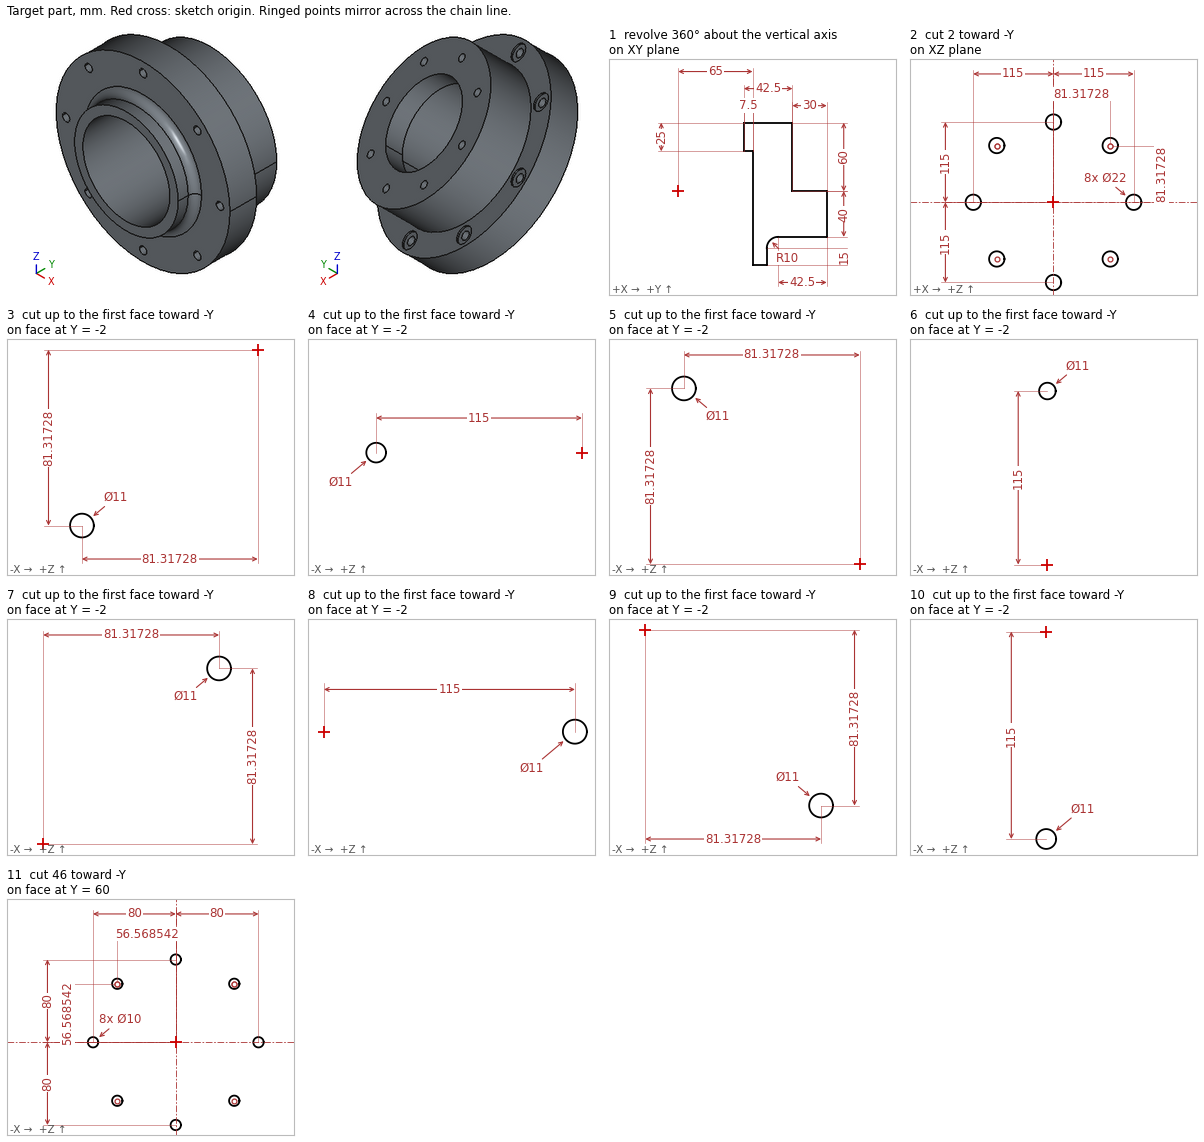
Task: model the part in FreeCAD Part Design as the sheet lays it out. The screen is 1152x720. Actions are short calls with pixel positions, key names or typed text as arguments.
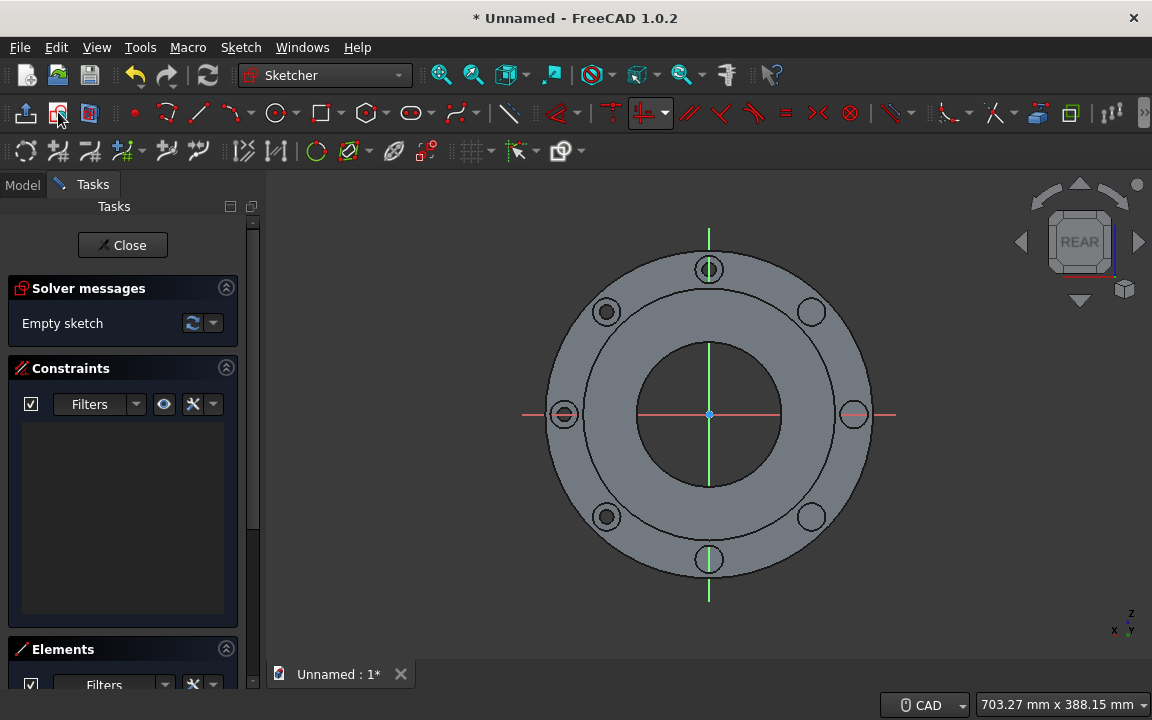
click(90, 114)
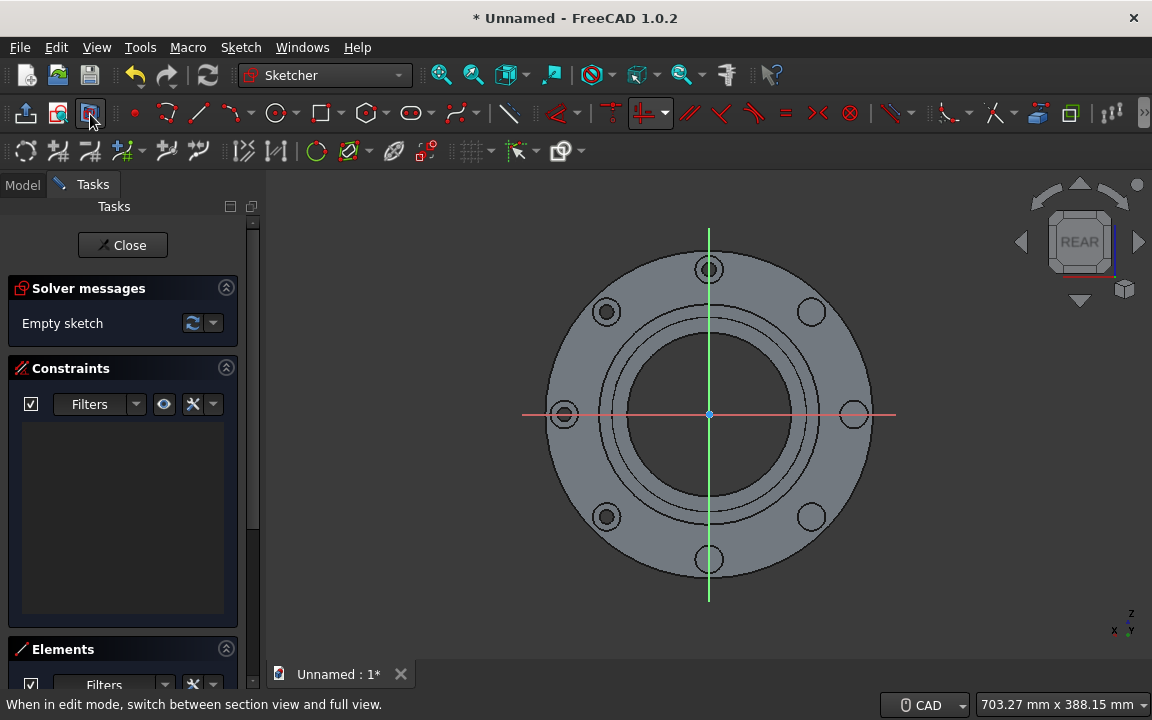
scroll(821, 307, up, 15)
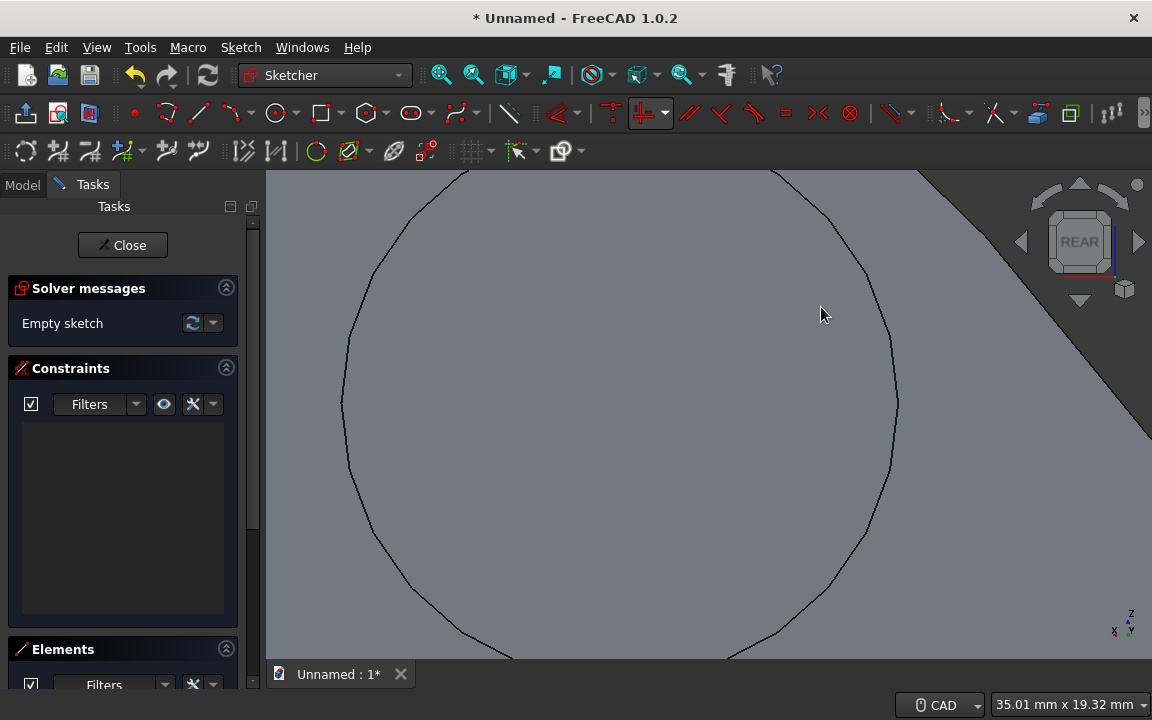
key(g)
key(c)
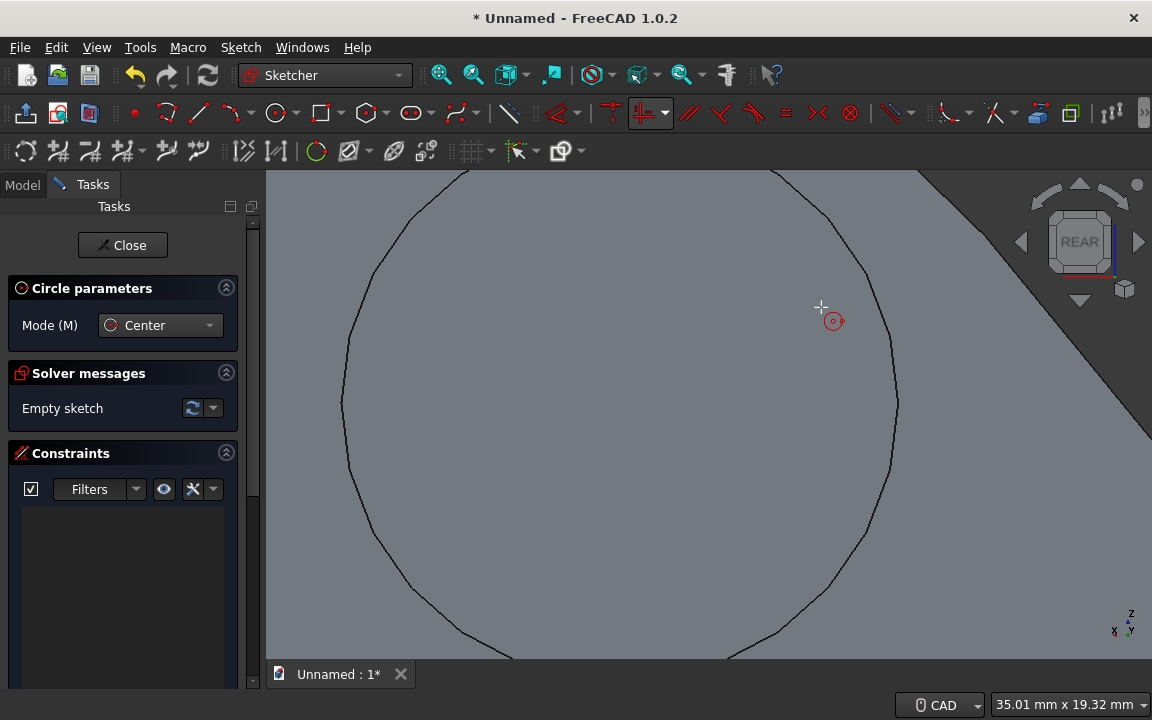
click(620, 403)
move(718, 305)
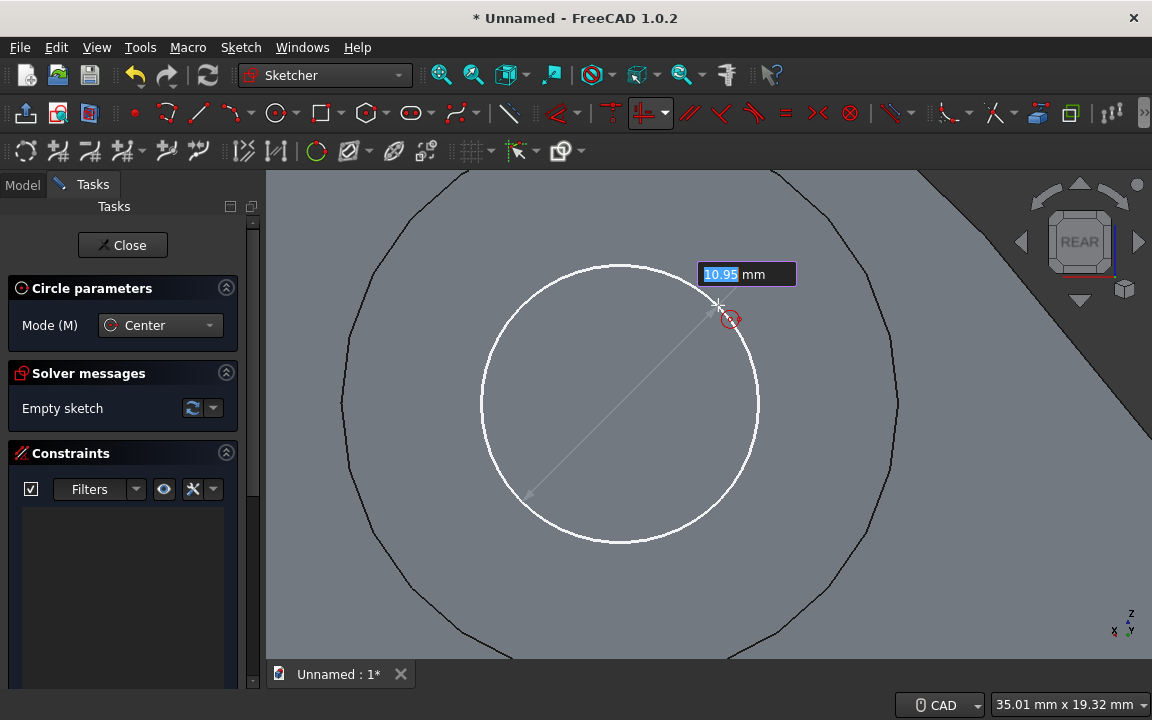
text(11)
key(Return)
key(Escape)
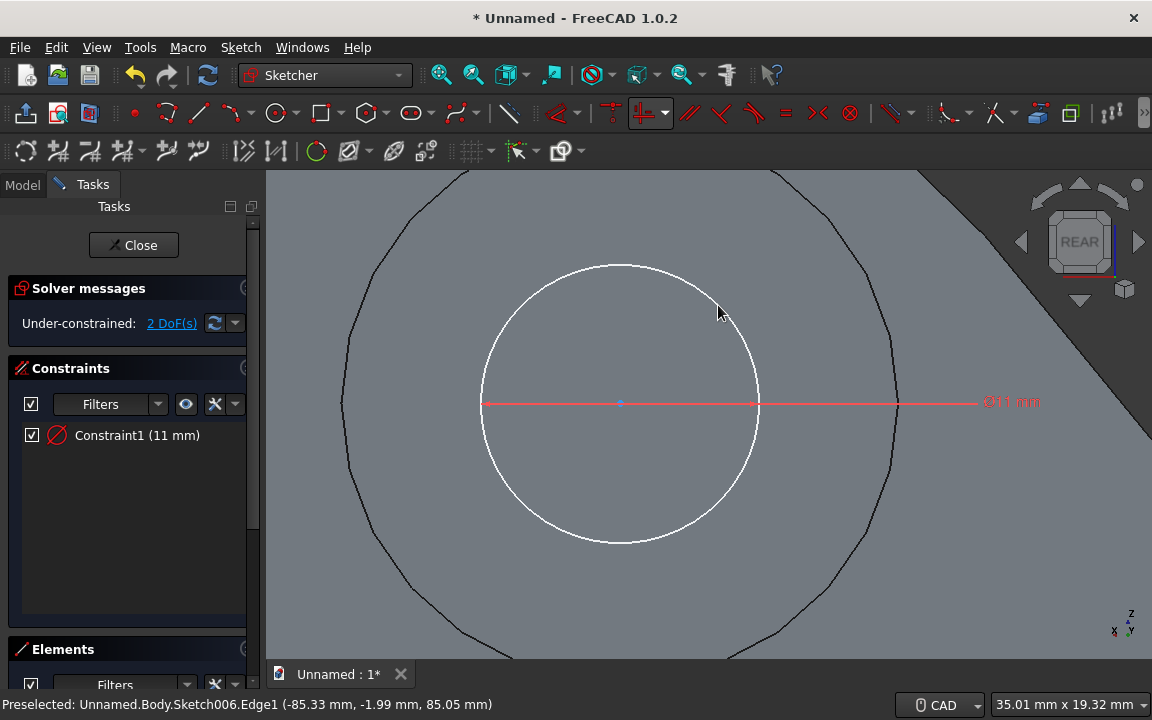
click(556, 114)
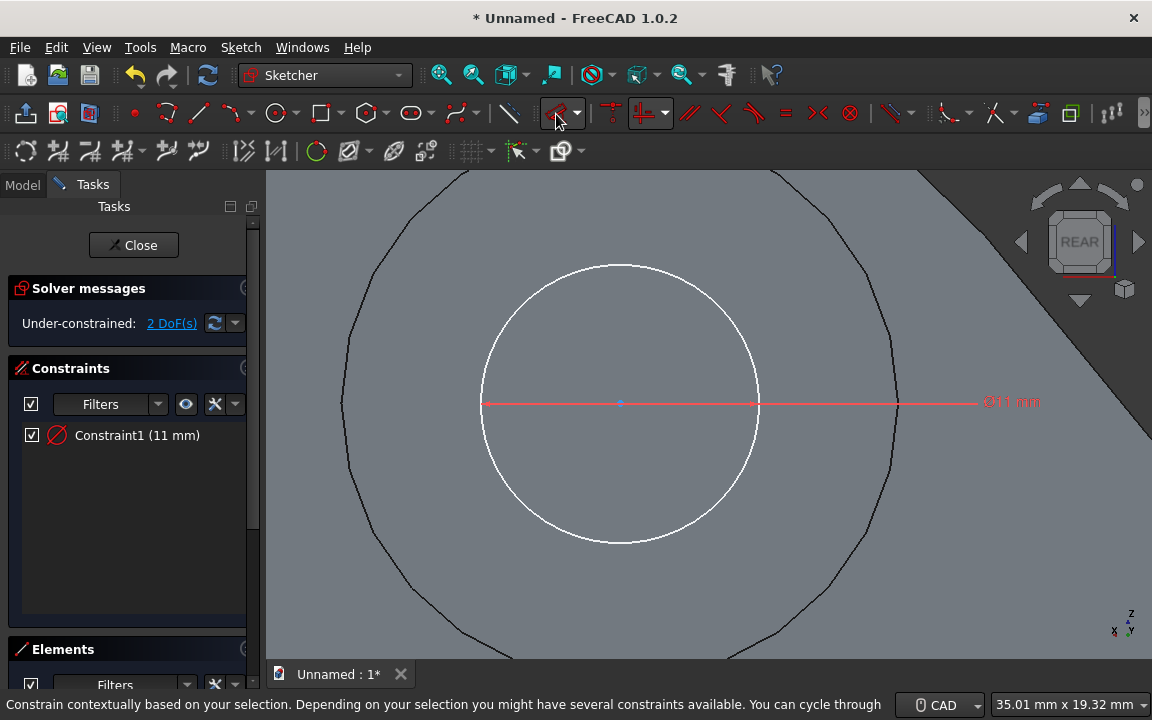
click(620, 404)
click(457, 370)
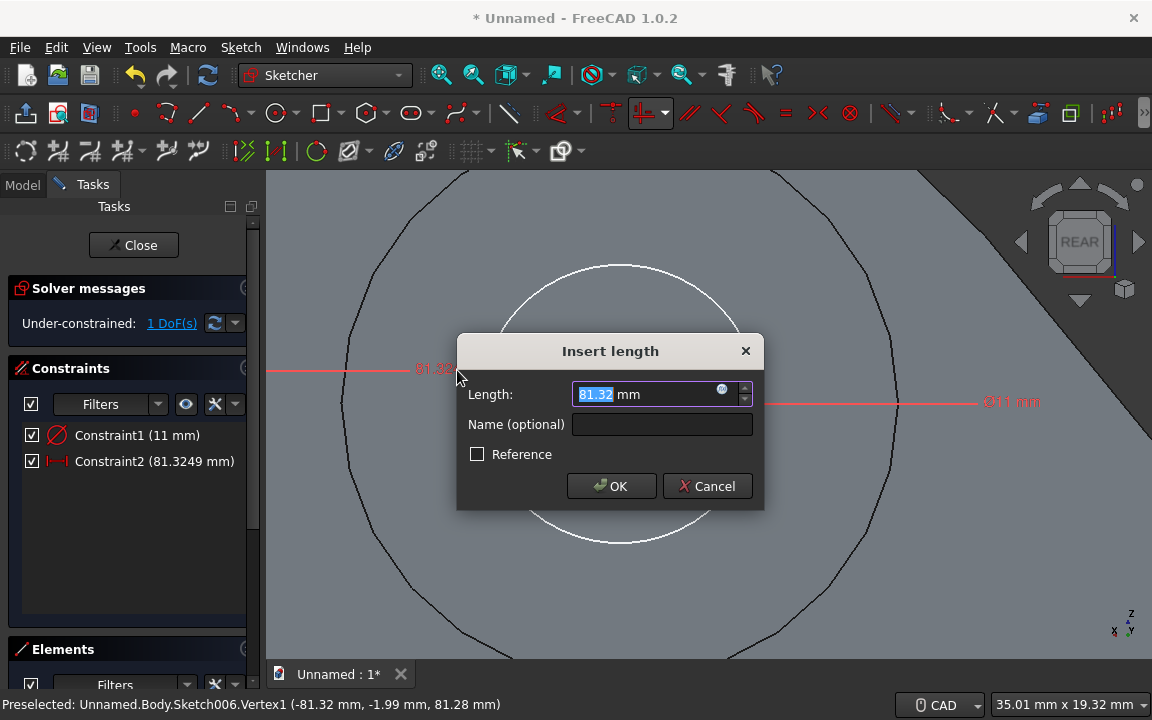
text(81.31728)
key(Return)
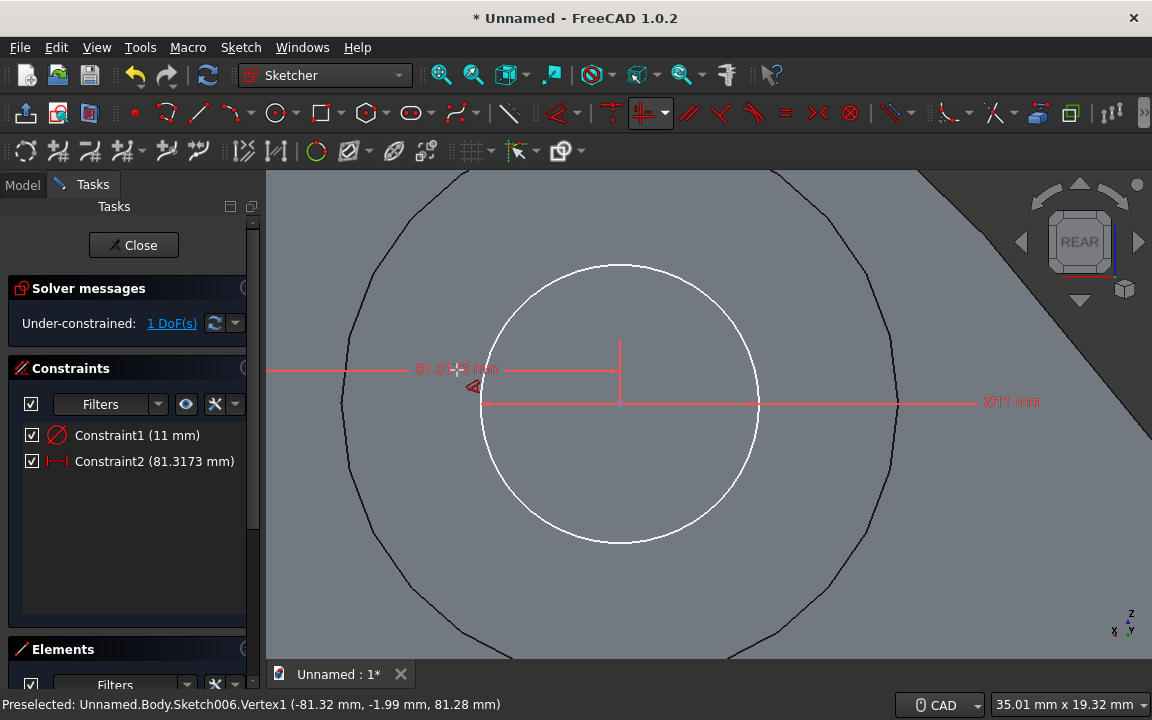
click(620, 404)
click(654, 518)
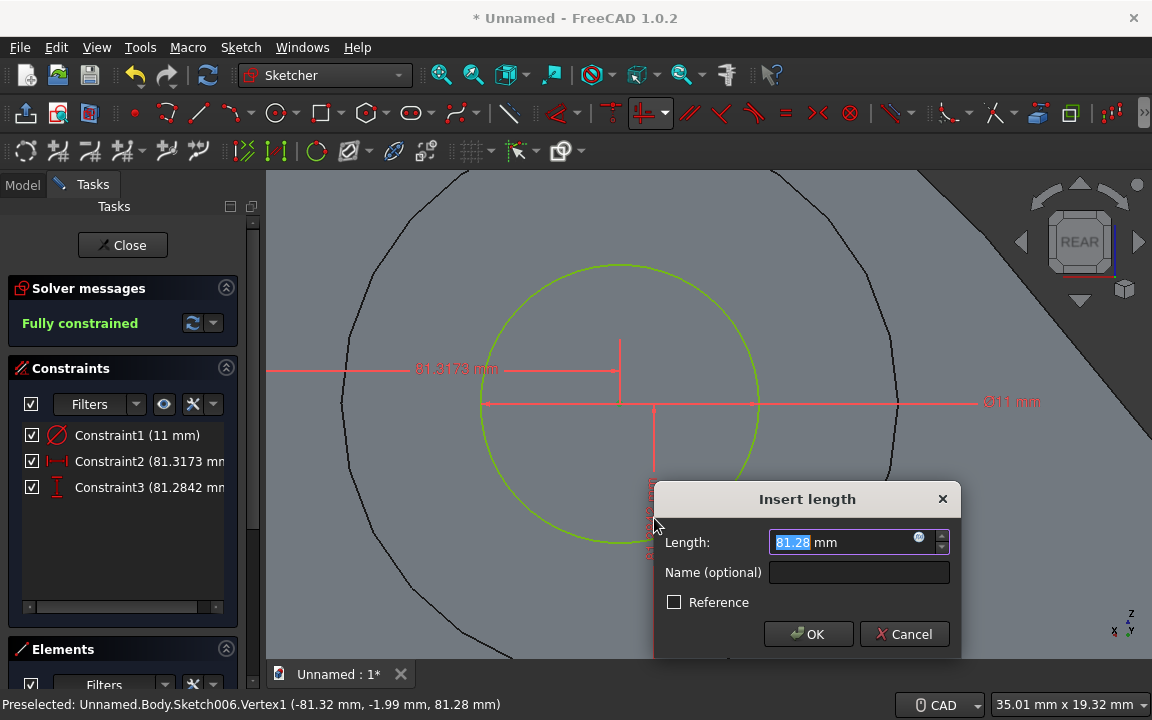
text(81.31728)
key(Return)
key(Escape)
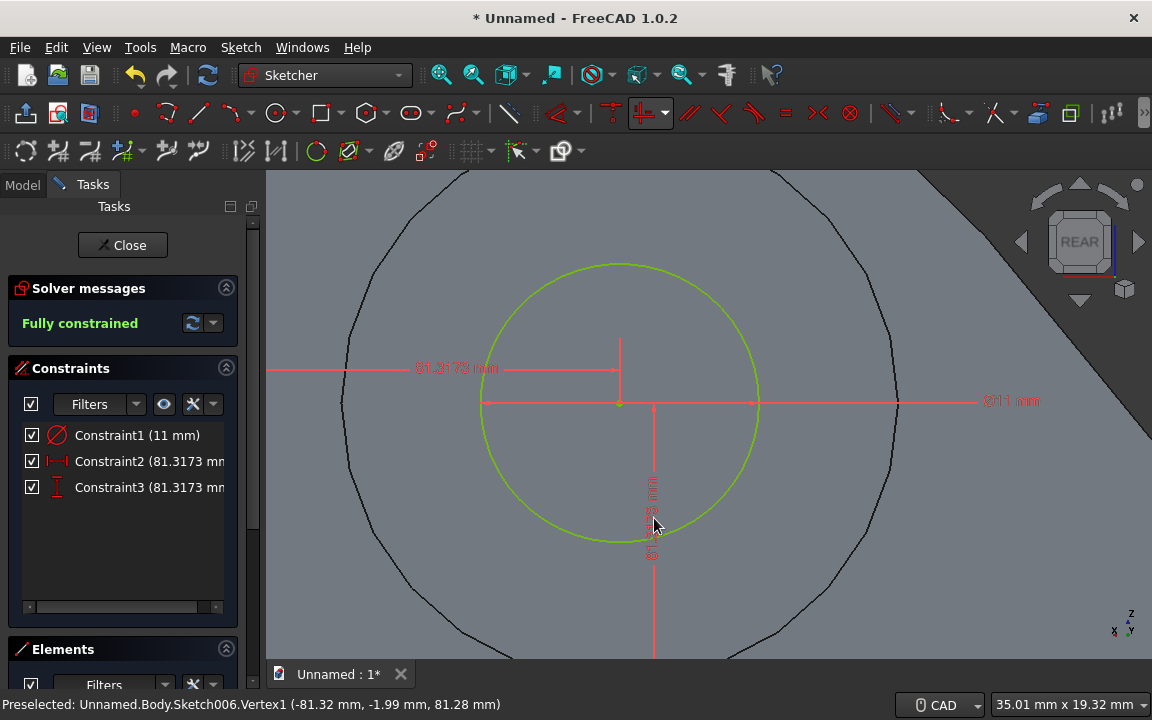
click(123, 245)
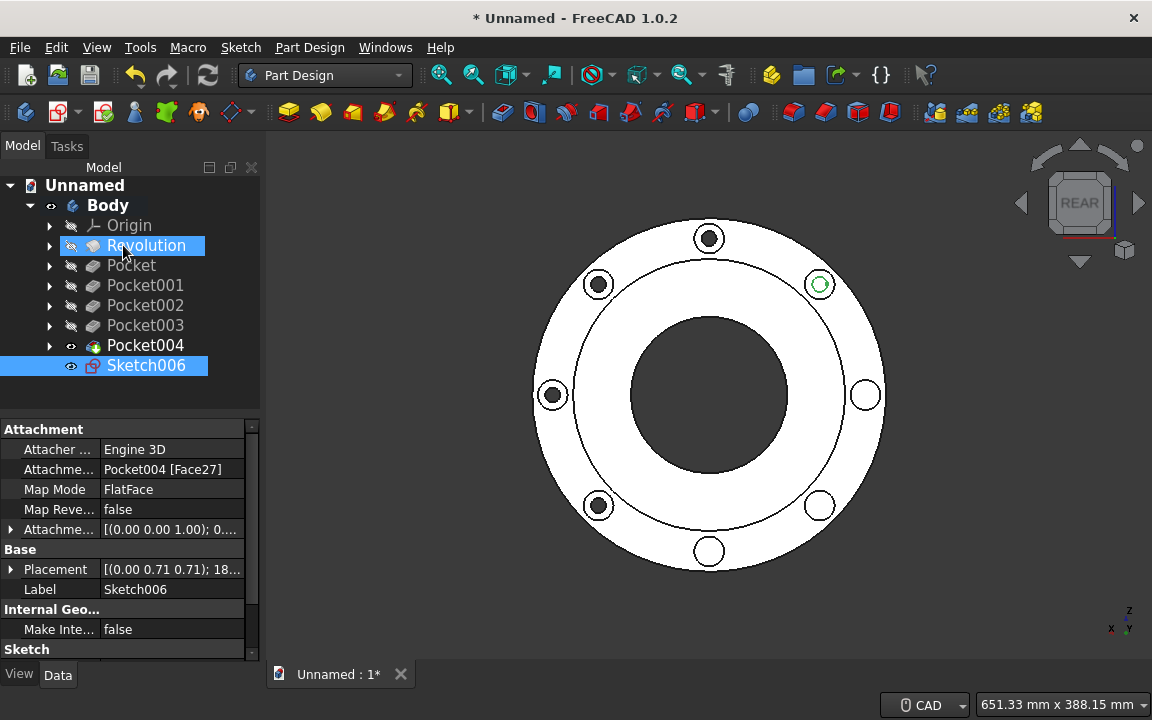
click(504, 112)